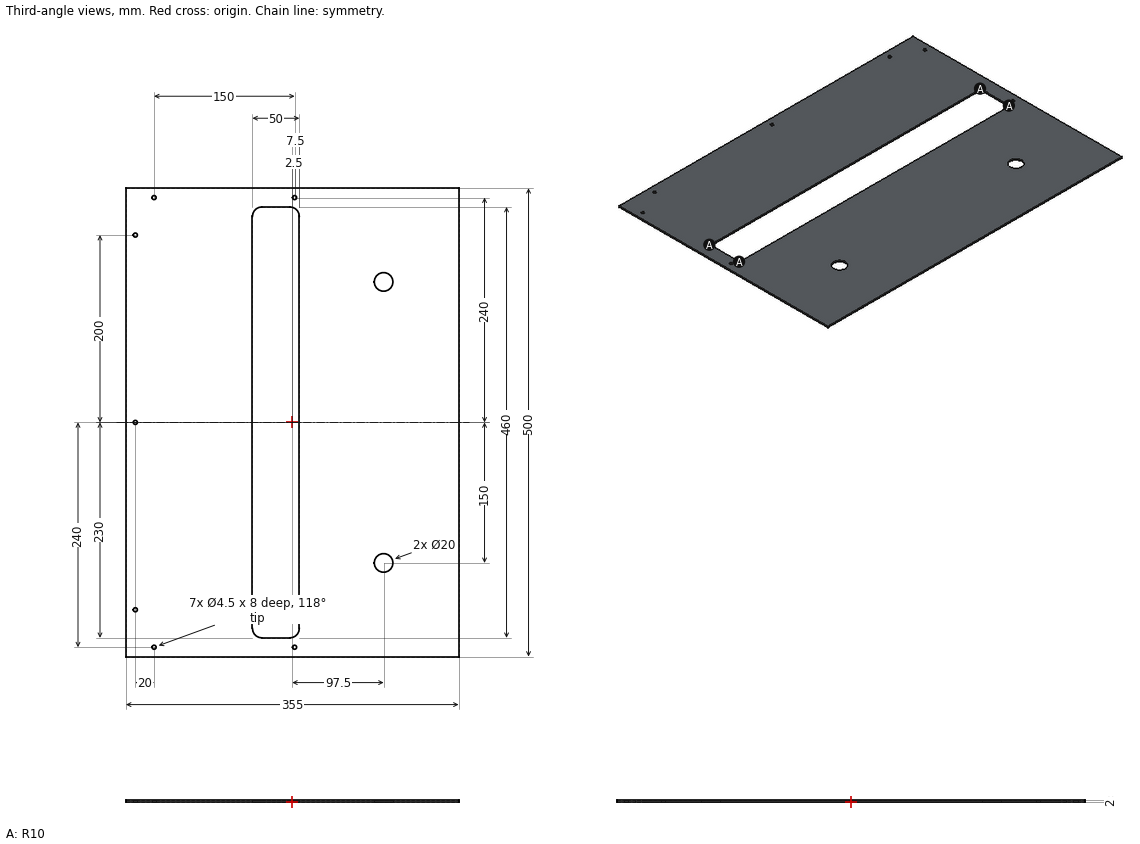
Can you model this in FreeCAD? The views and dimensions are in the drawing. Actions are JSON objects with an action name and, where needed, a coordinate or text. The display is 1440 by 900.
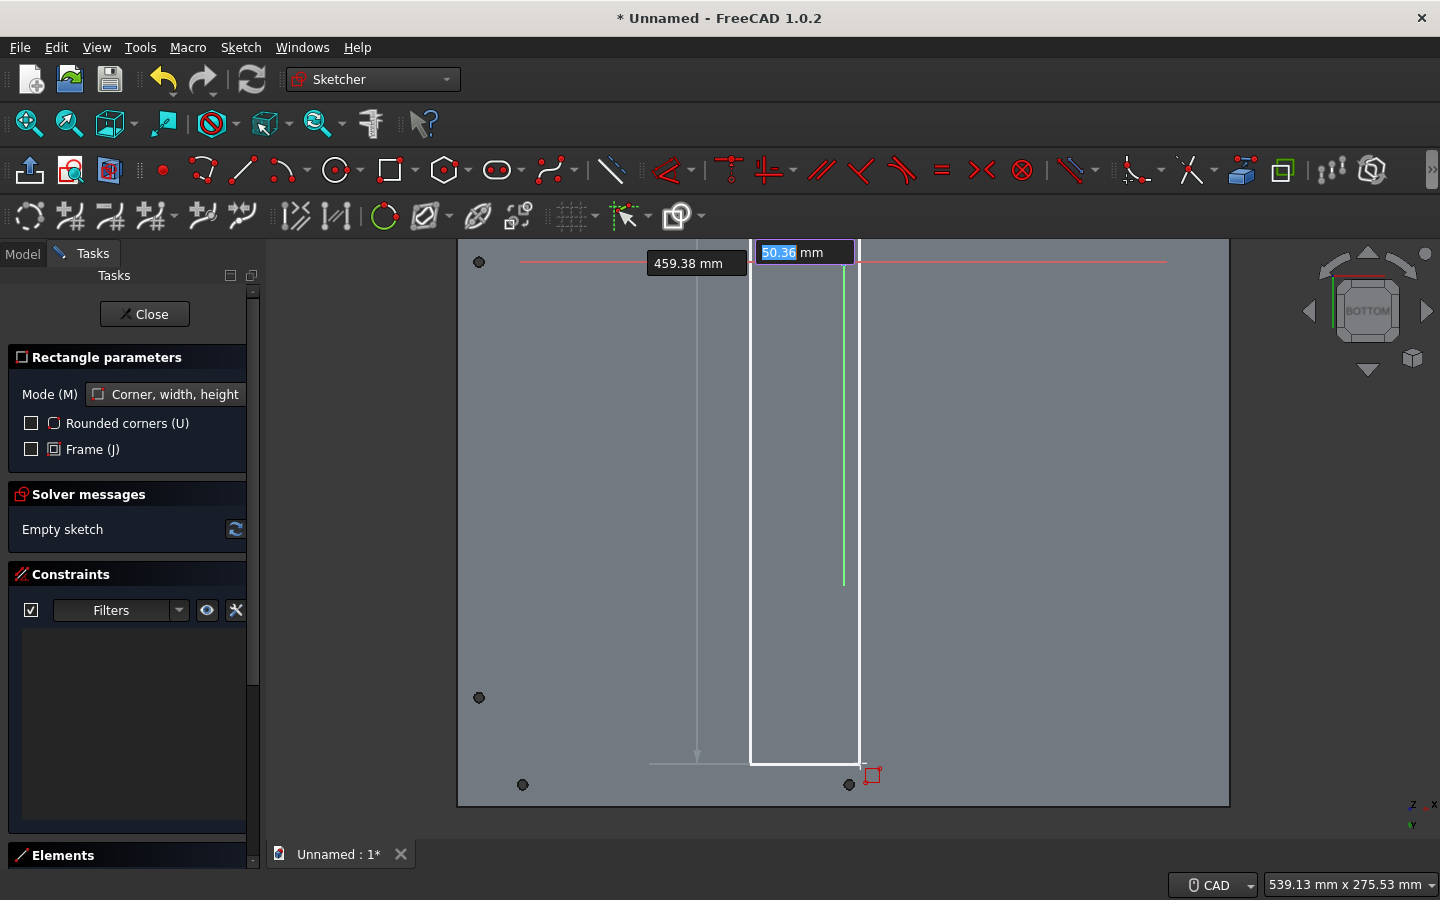
{"action": "type", "text": "50"}
{"action": "key", "text": "Tab"}
{"action": "type", "text": "460"}
{"action": "key", "text": "Return"}
{"action": "key", "text": "Escape"}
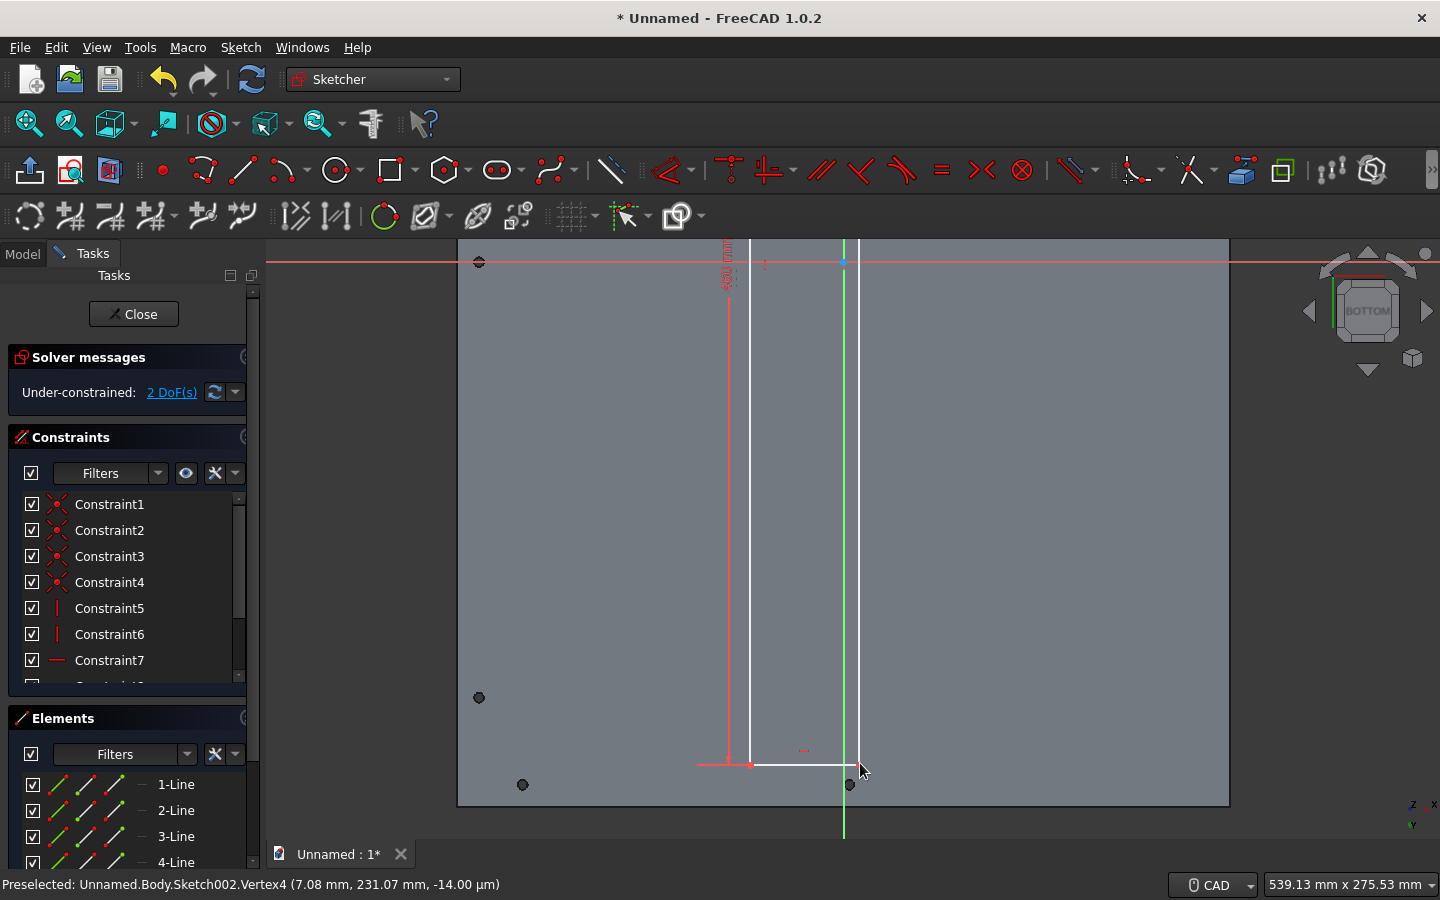
{"action": "left_click", "coordinate": [666, 170]}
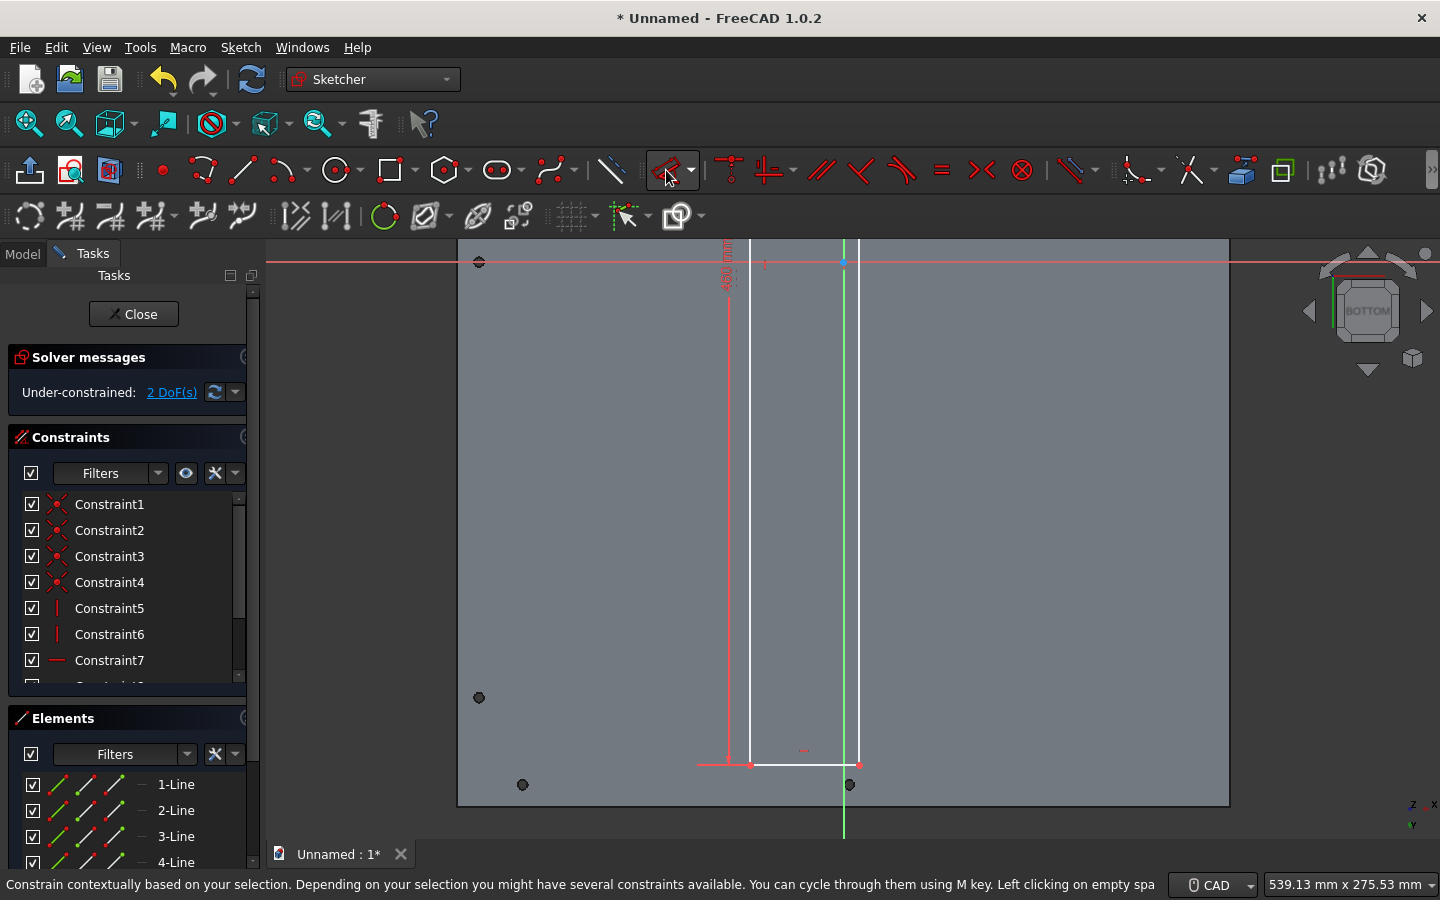
{"action": "scroll", "coordinate": [772, 700], "scroll_direction": "down", "scroll_amount": 5}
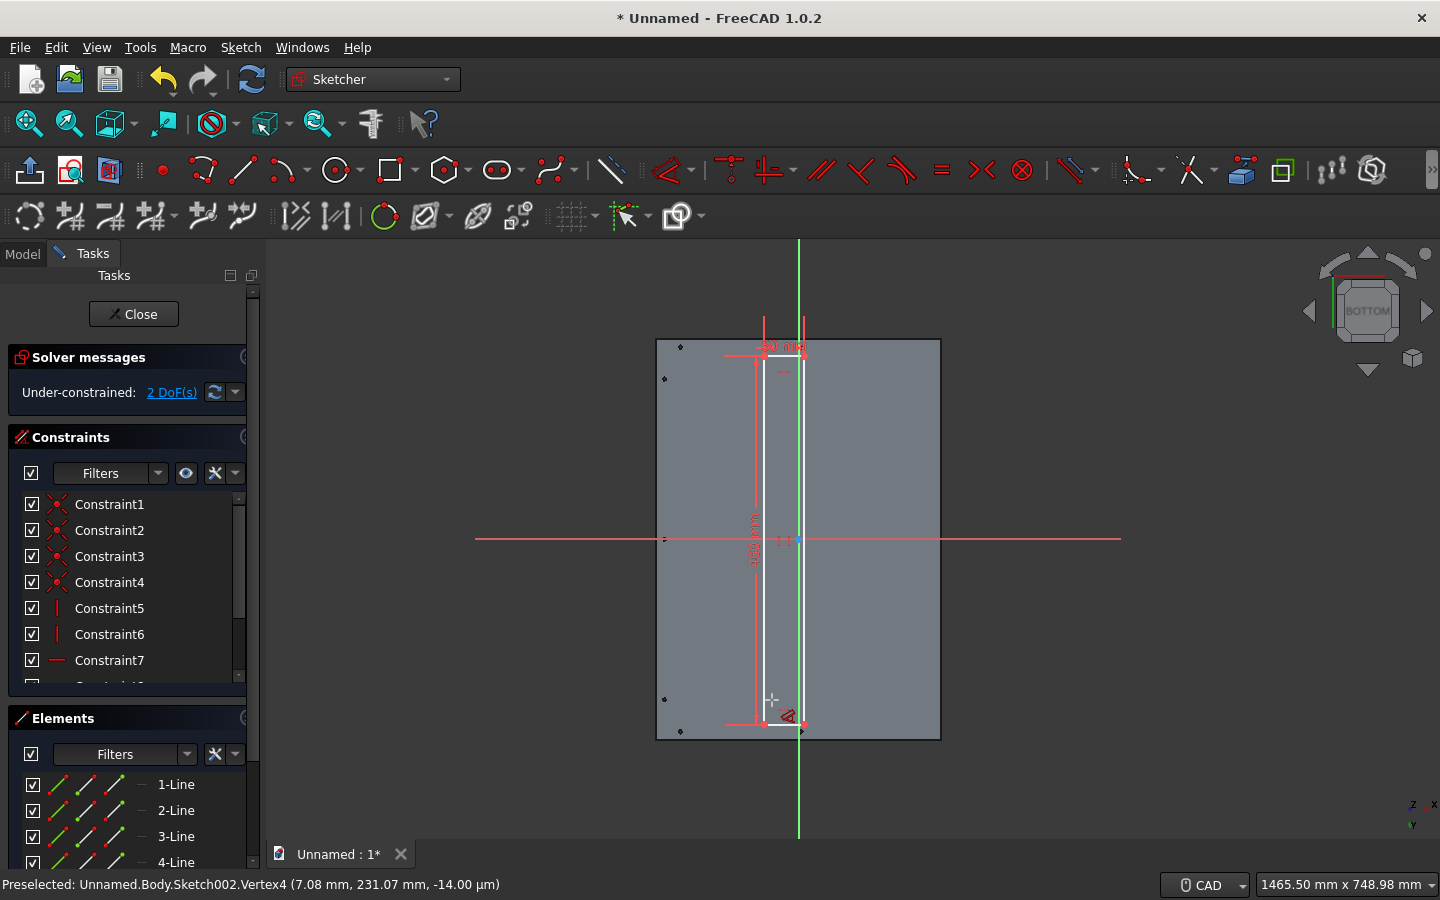
{"action": "left_click", "coordinate": [764, 356]}
{"action": "left_click", "coordinate": [730, 448]}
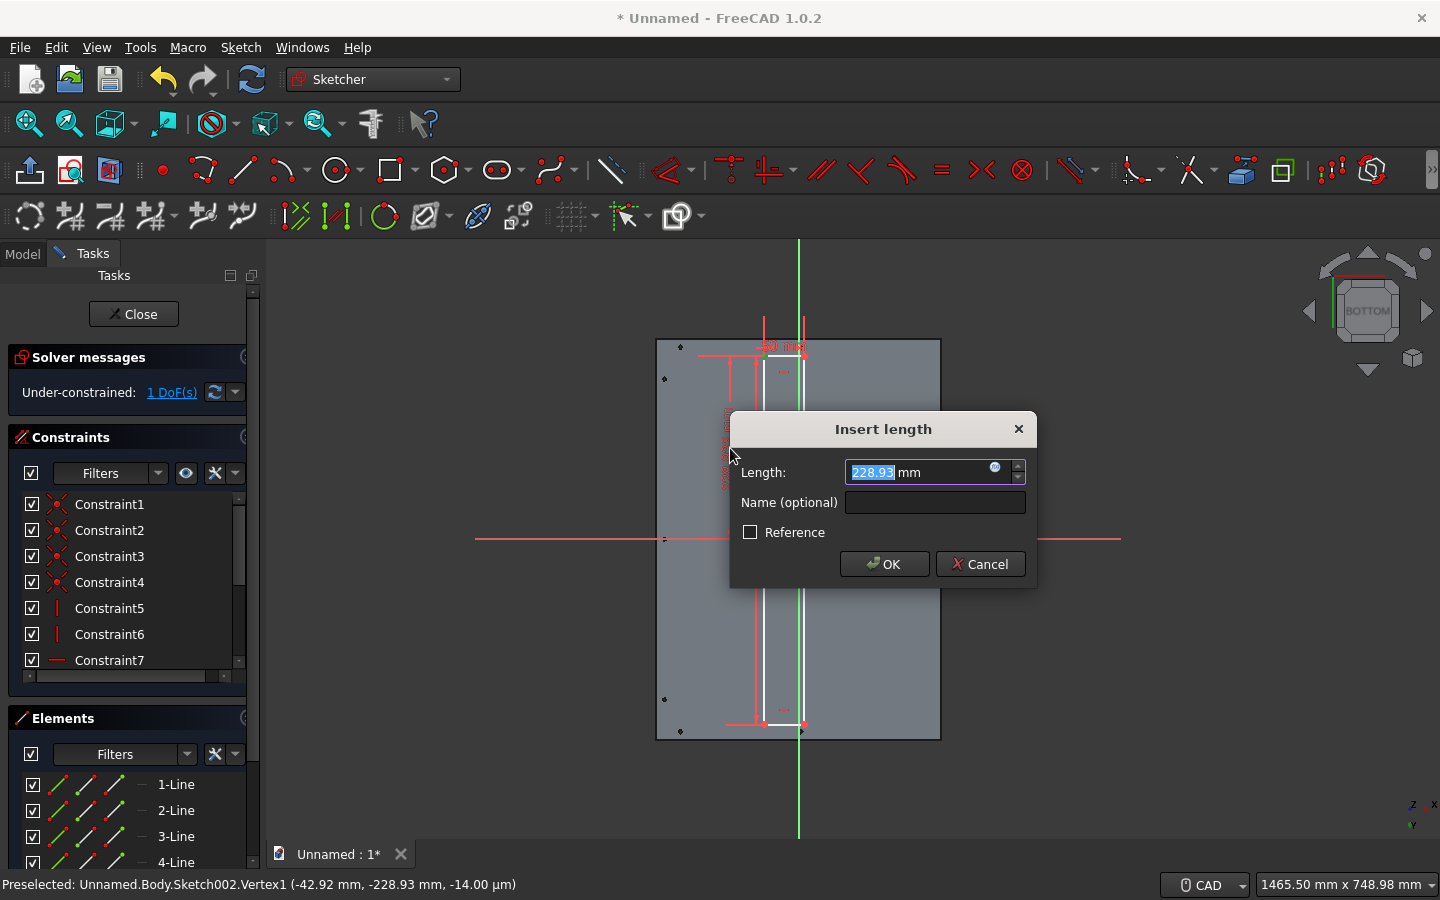
{"action": "type", "text": "230"}
{"action": "key", "text": "Return"}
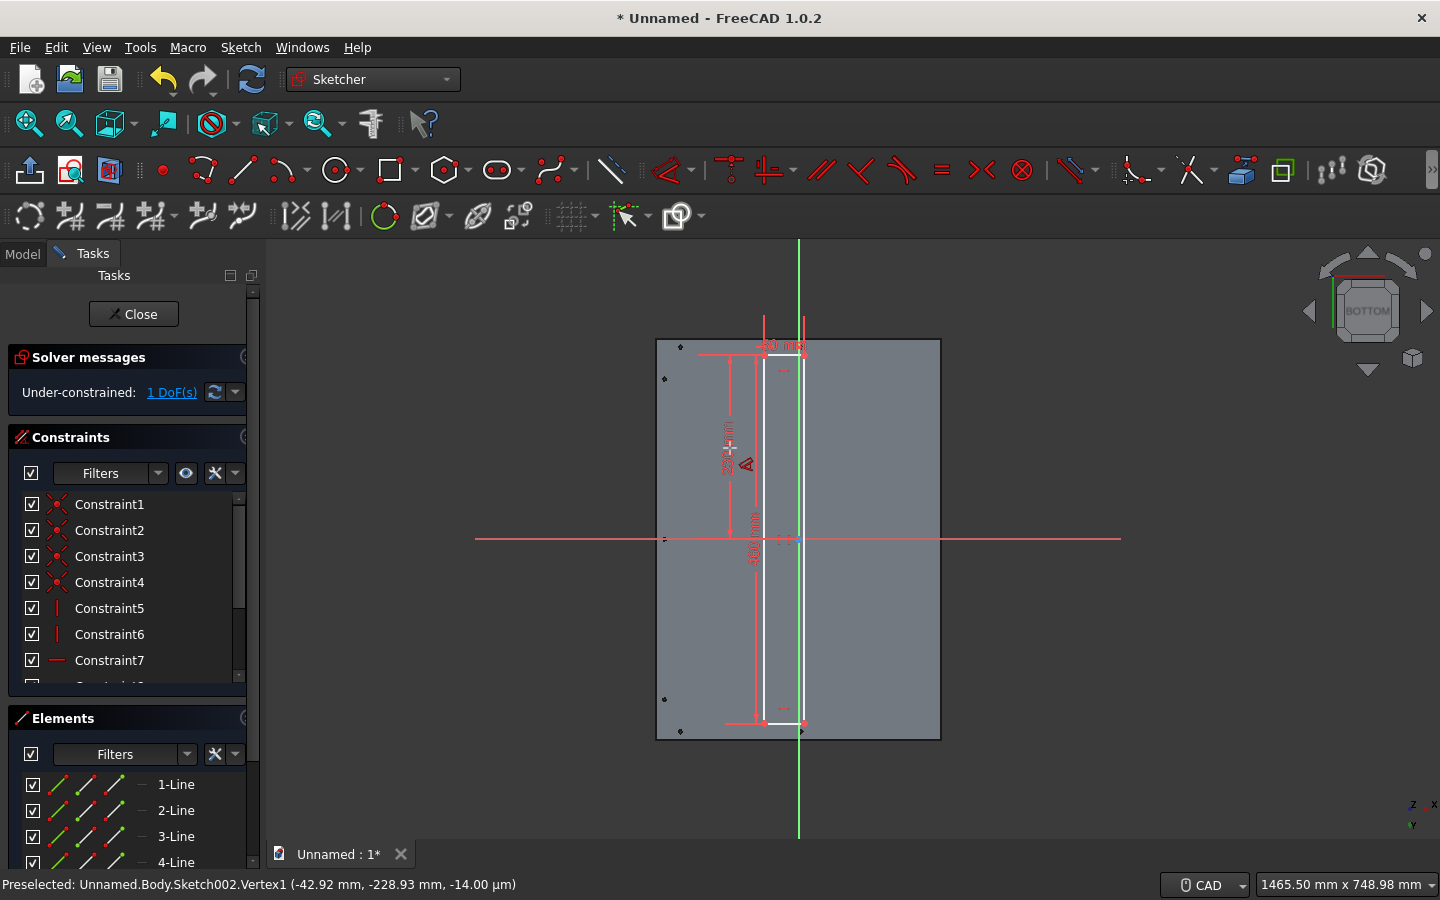
{"action": "scroll", "coordinate": [804, 724], "scroll_direction": "up", "scroll_amount": 10}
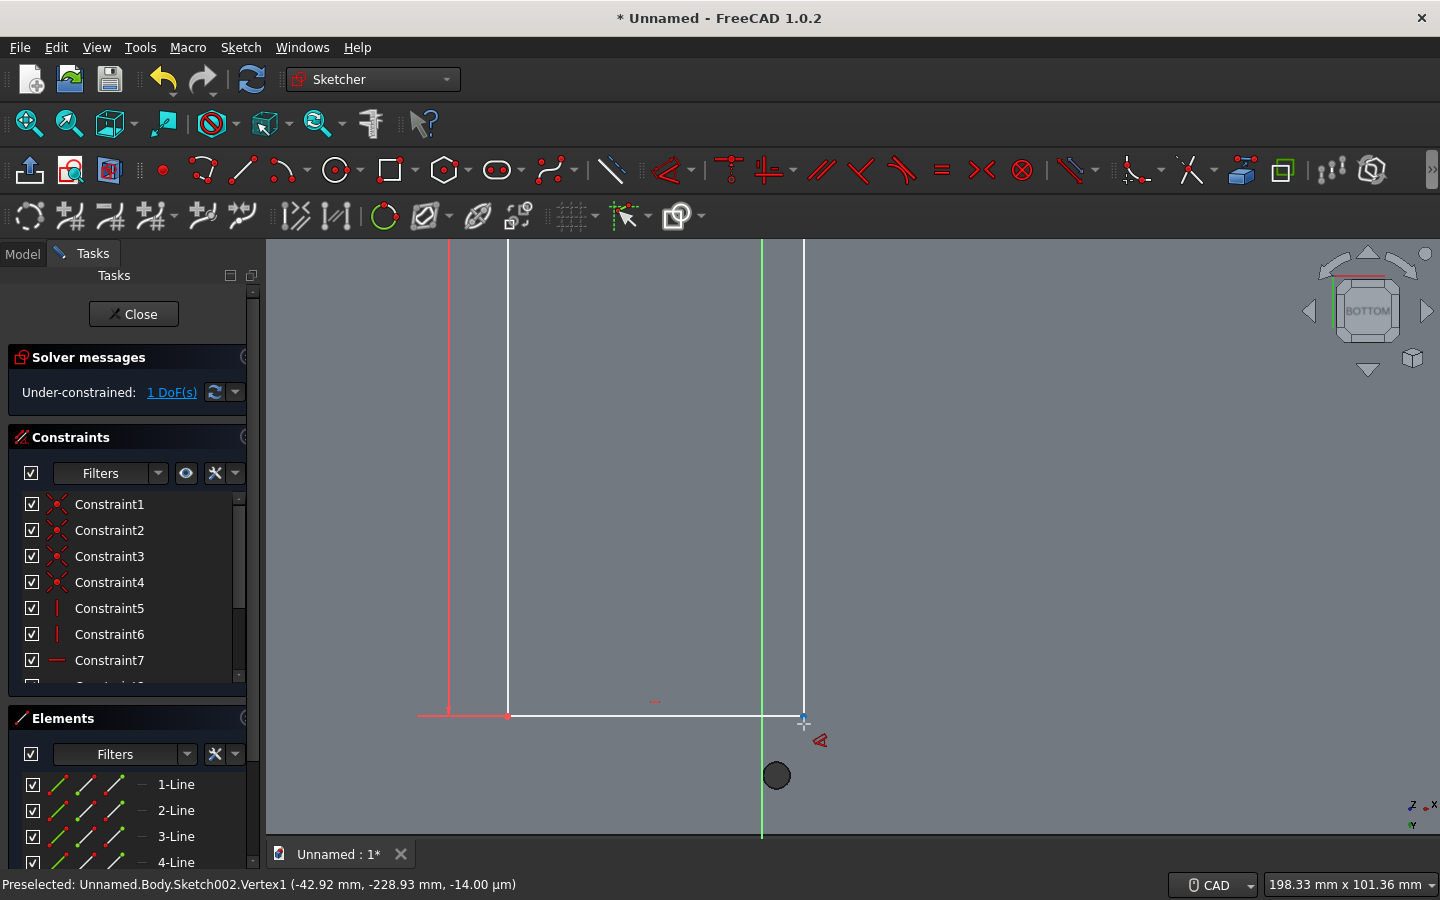
{"action": "left_click", "coordinate": [804, 716]}
{"action": "left_click", "coordinate": [783, 750]}